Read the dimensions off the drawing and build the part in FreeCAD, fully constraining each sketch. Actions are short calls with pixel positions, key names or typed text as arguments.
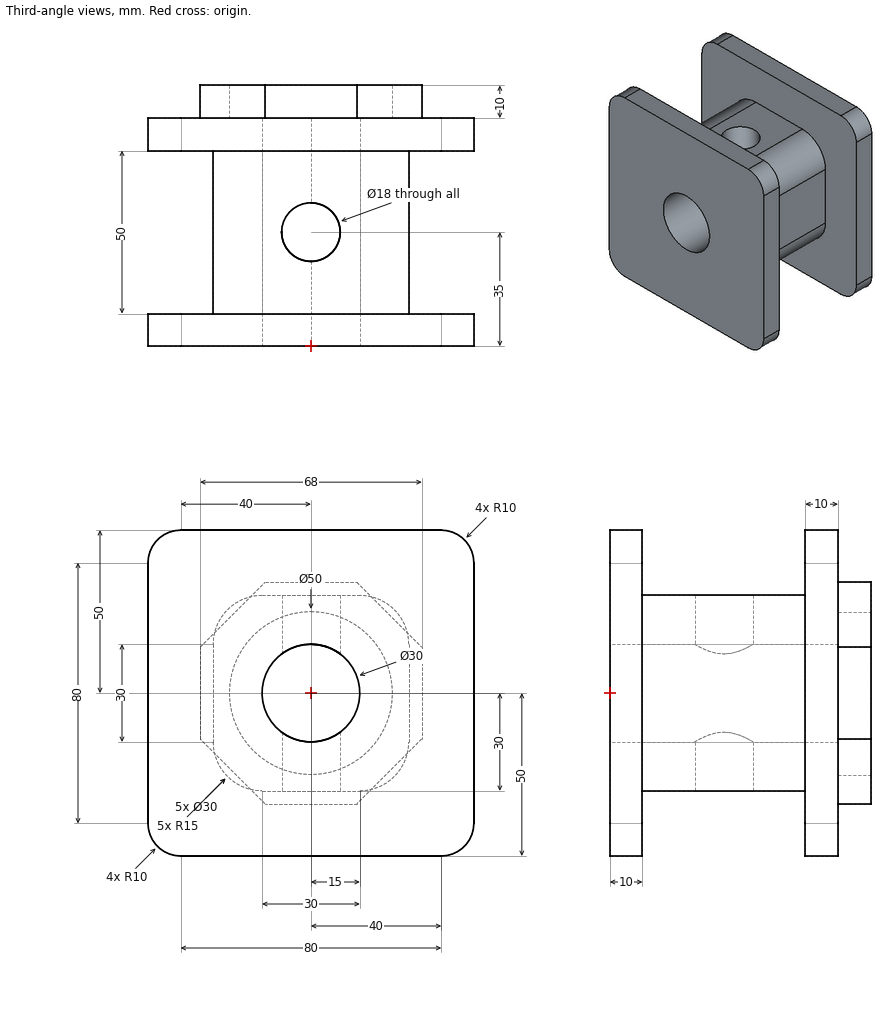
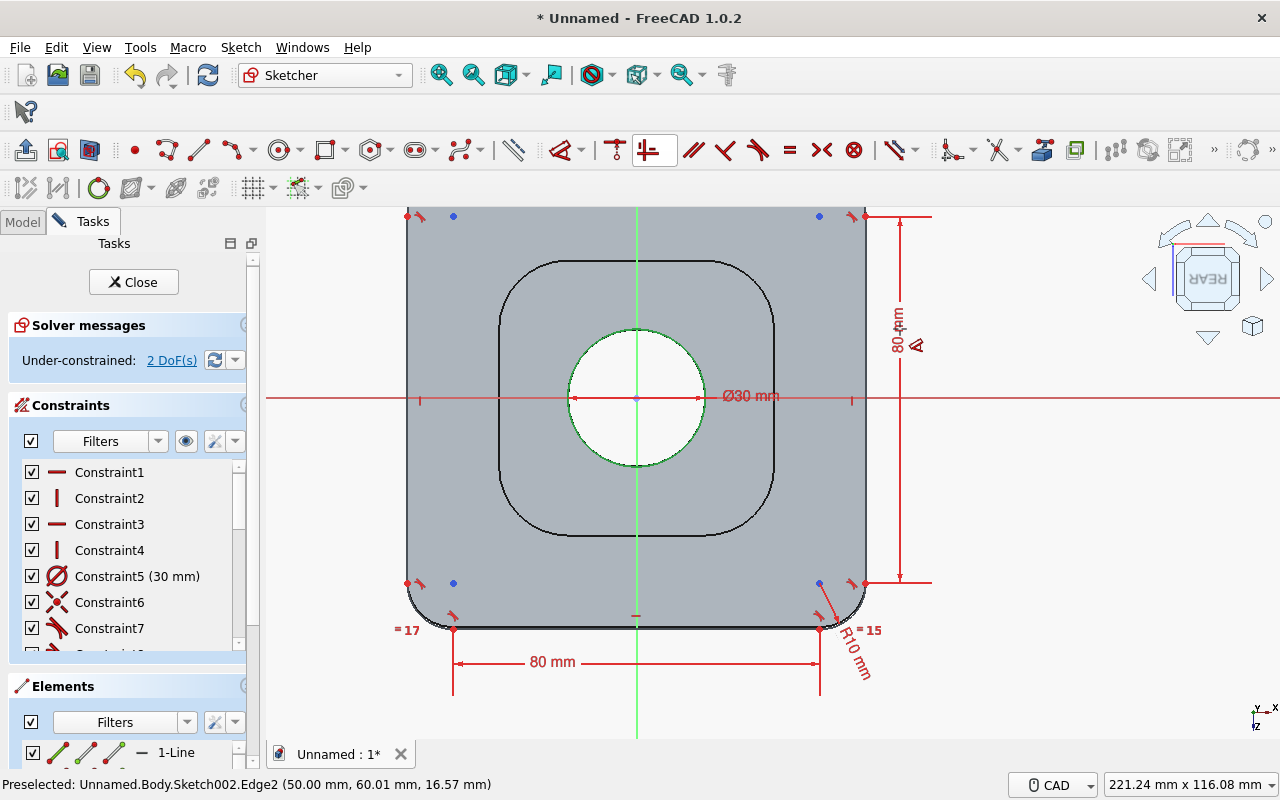
click(453, 629)
click(481, 663)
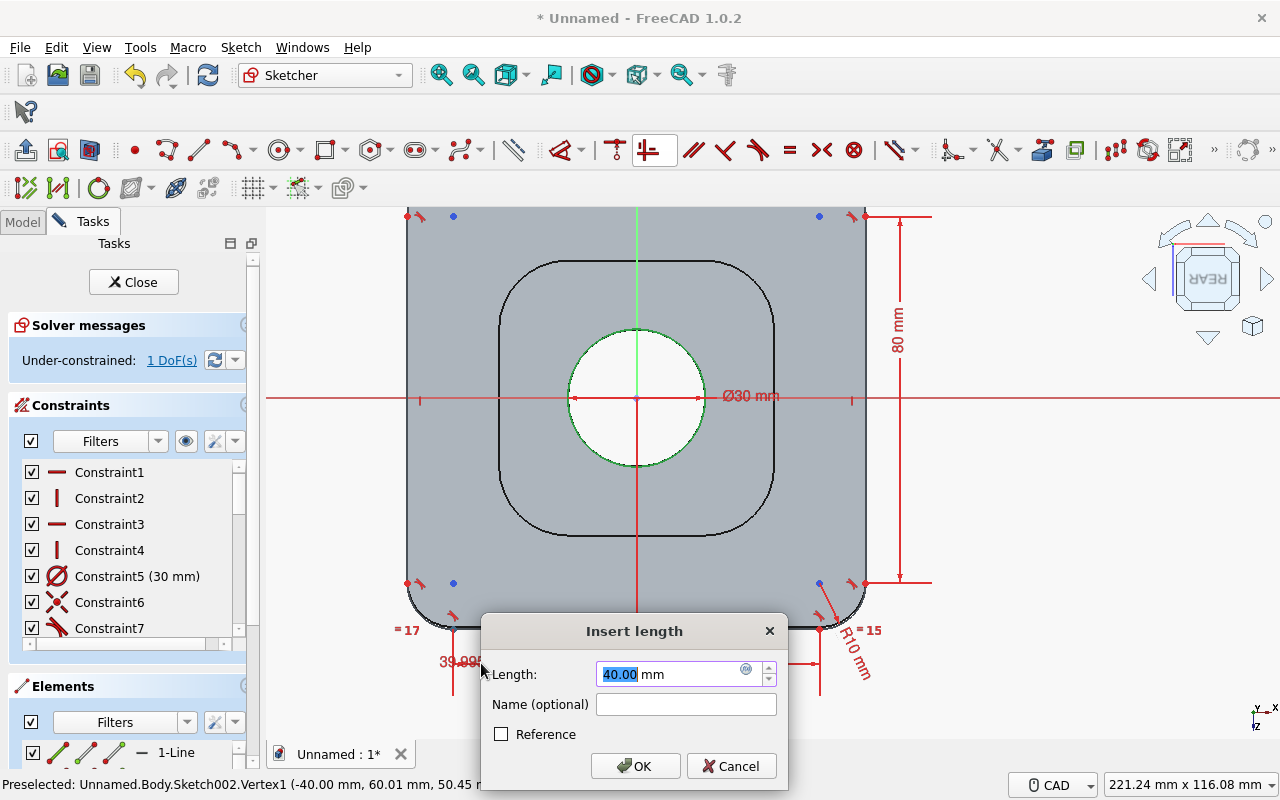
text(40)
key(Return)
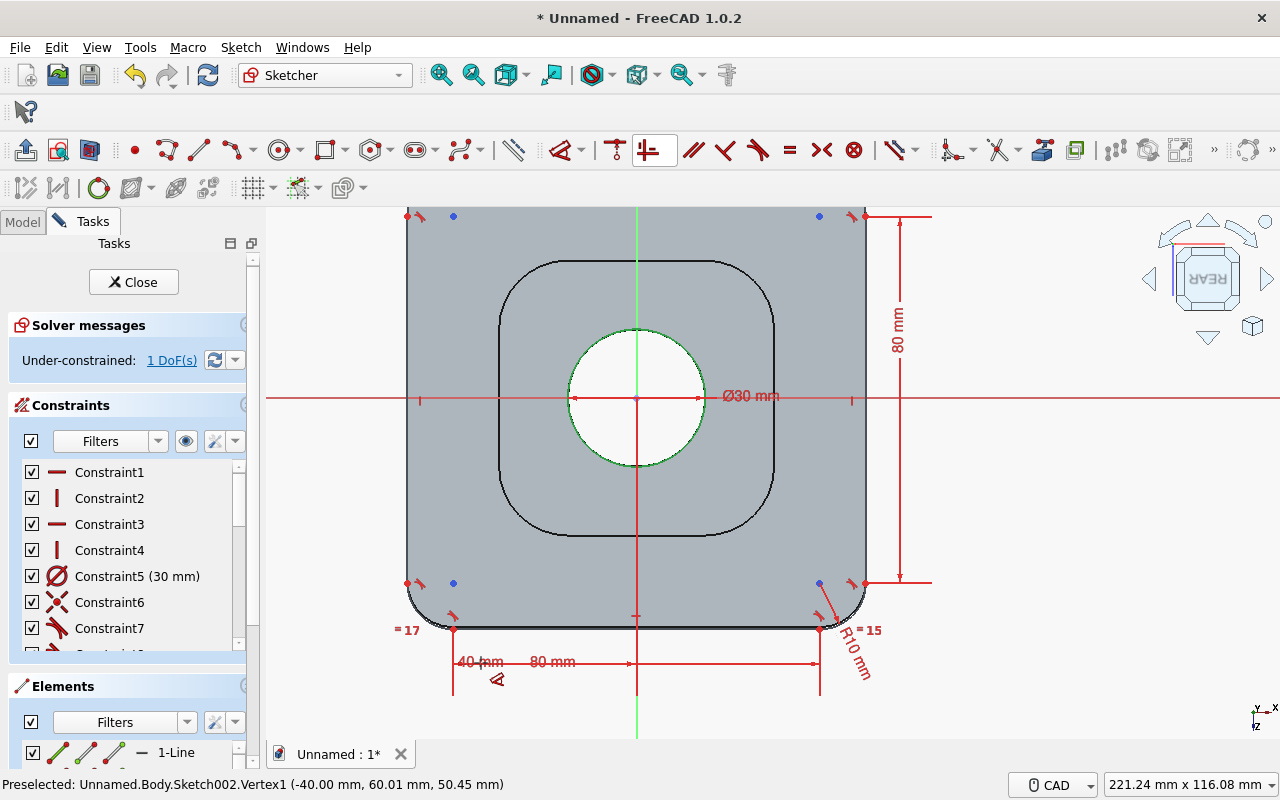
click(453, 629)
click(671, 514)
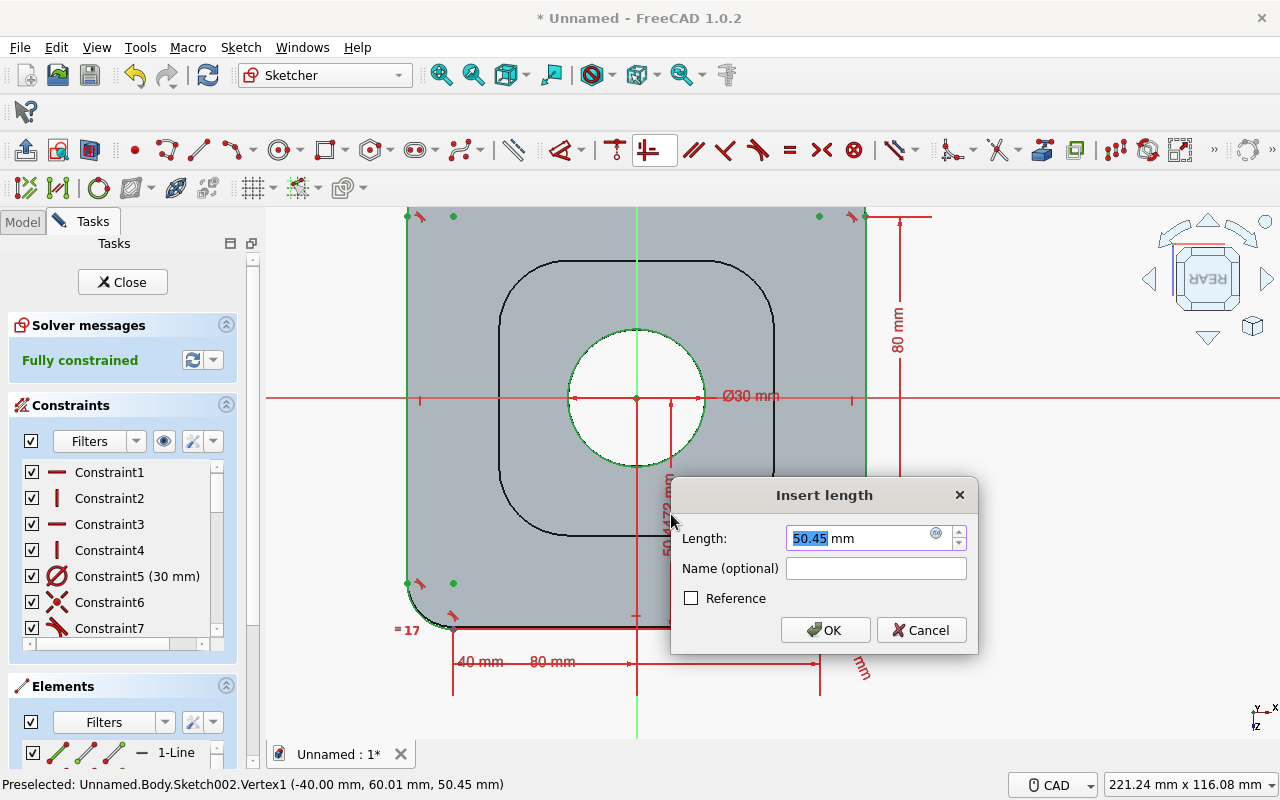
text(50)
key(Return)
key(Escape)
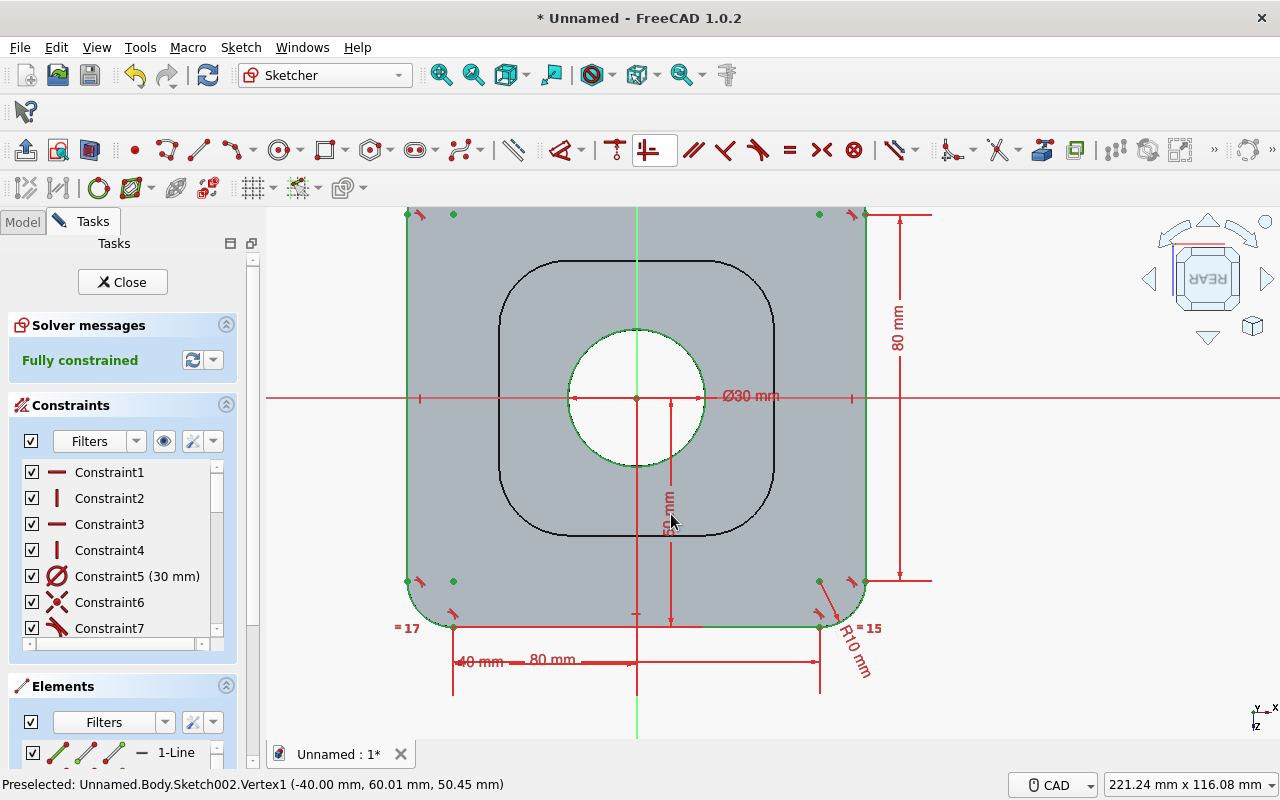
click(123, 282)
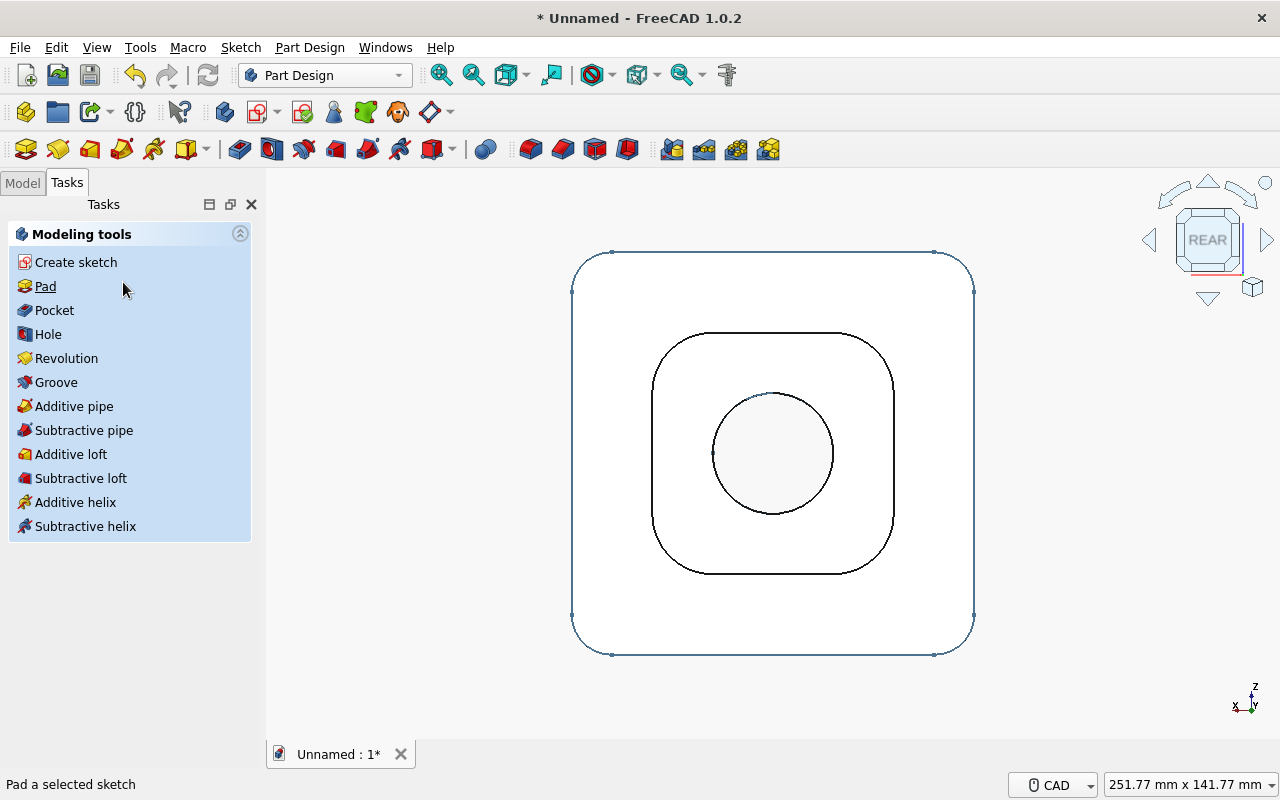
click(26, 150)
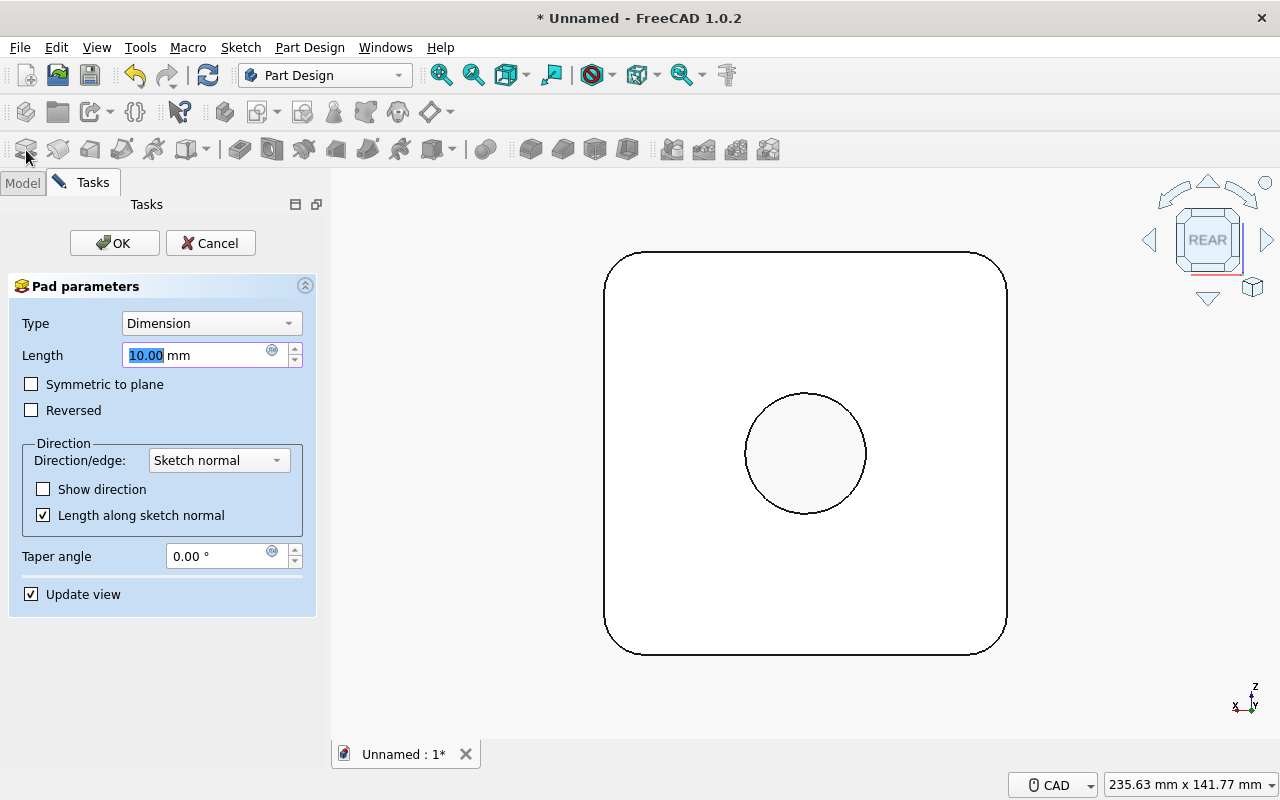
text(10)
key(Tab)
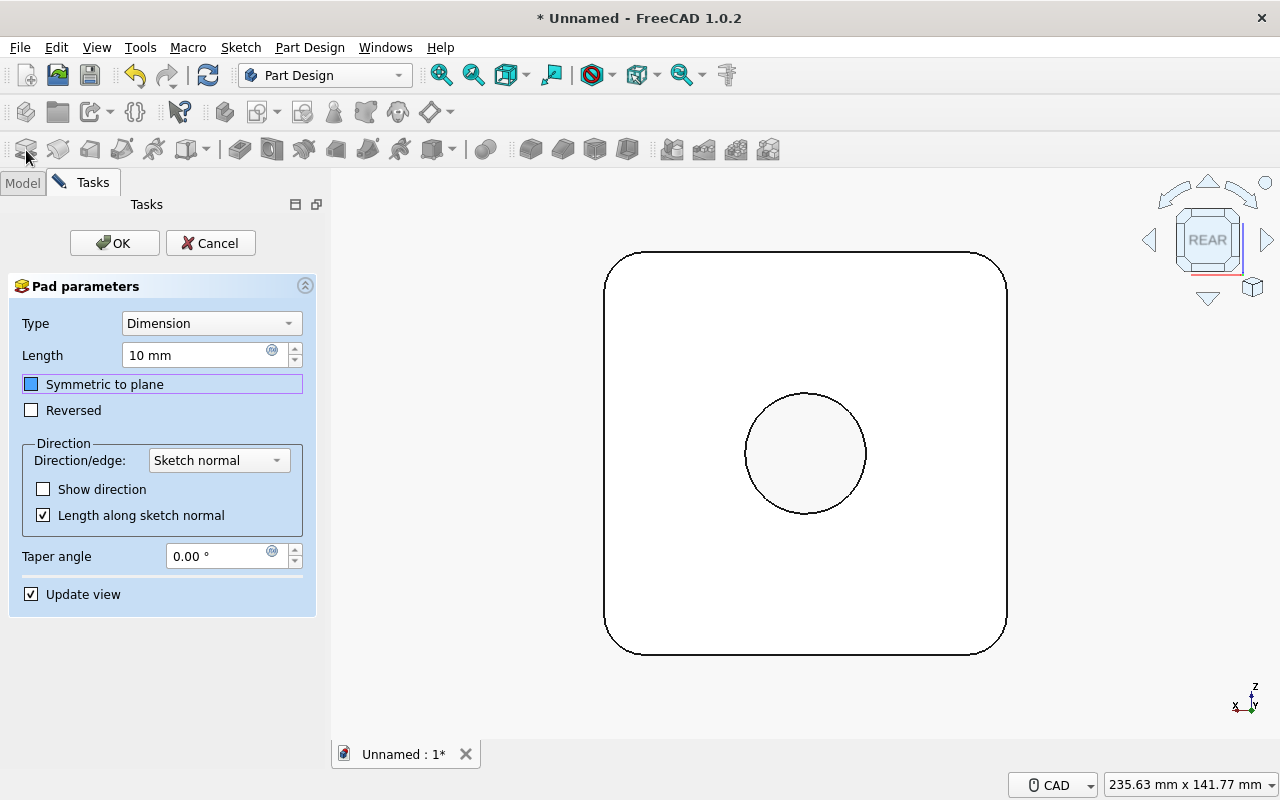
click(115, 243)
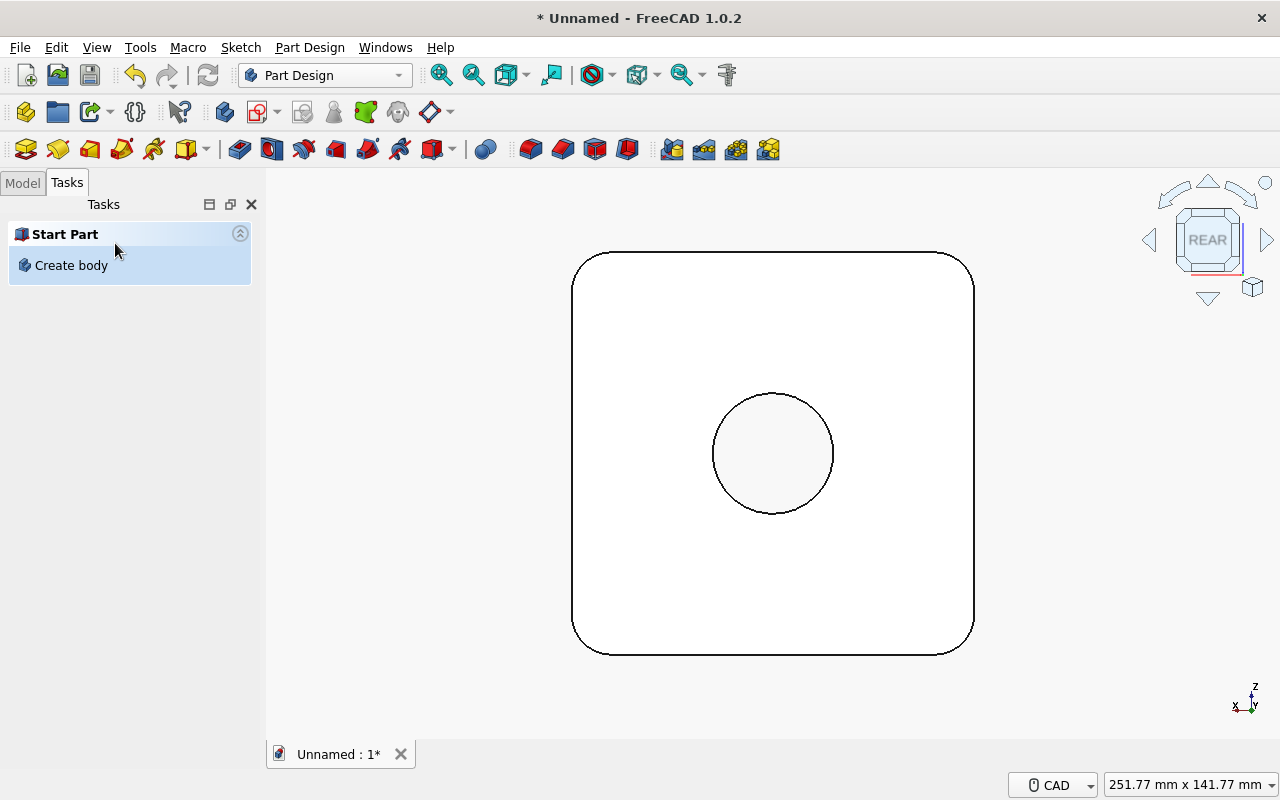
click(658, 568)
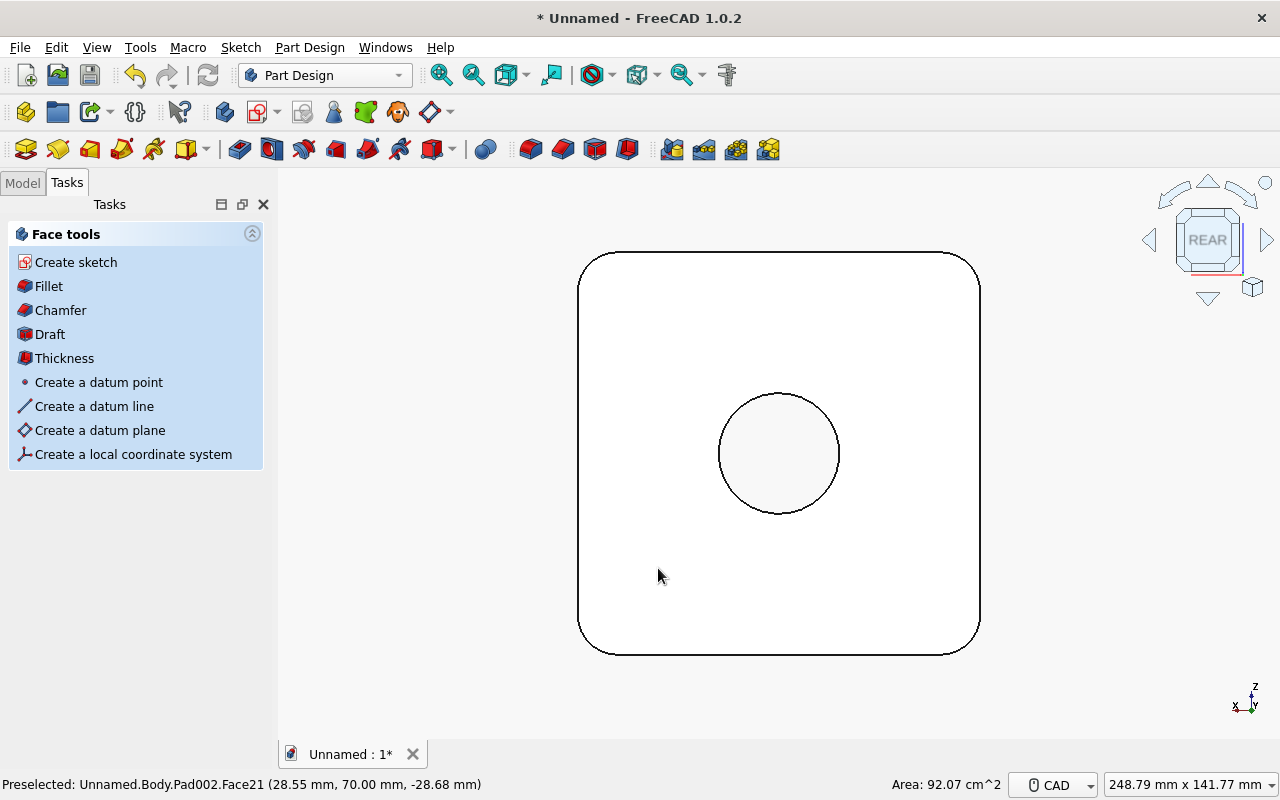
click(258, 112)